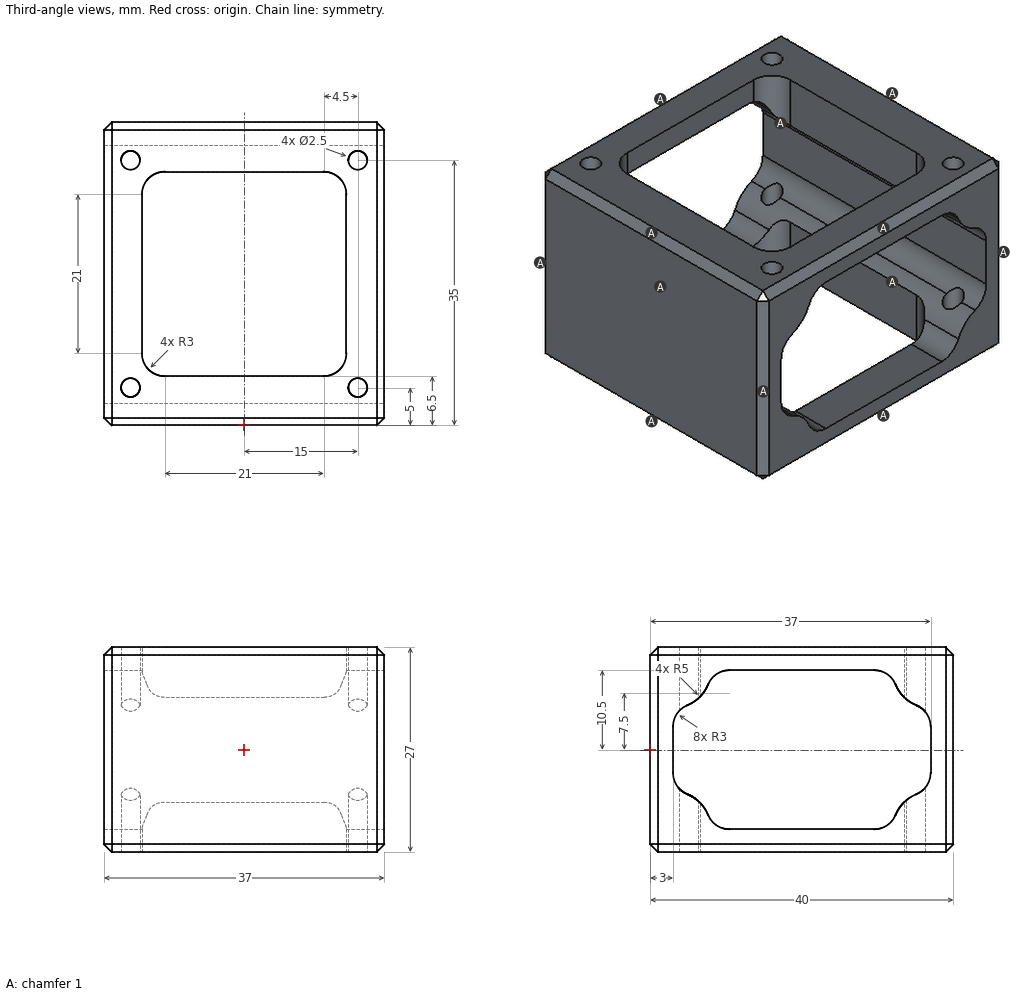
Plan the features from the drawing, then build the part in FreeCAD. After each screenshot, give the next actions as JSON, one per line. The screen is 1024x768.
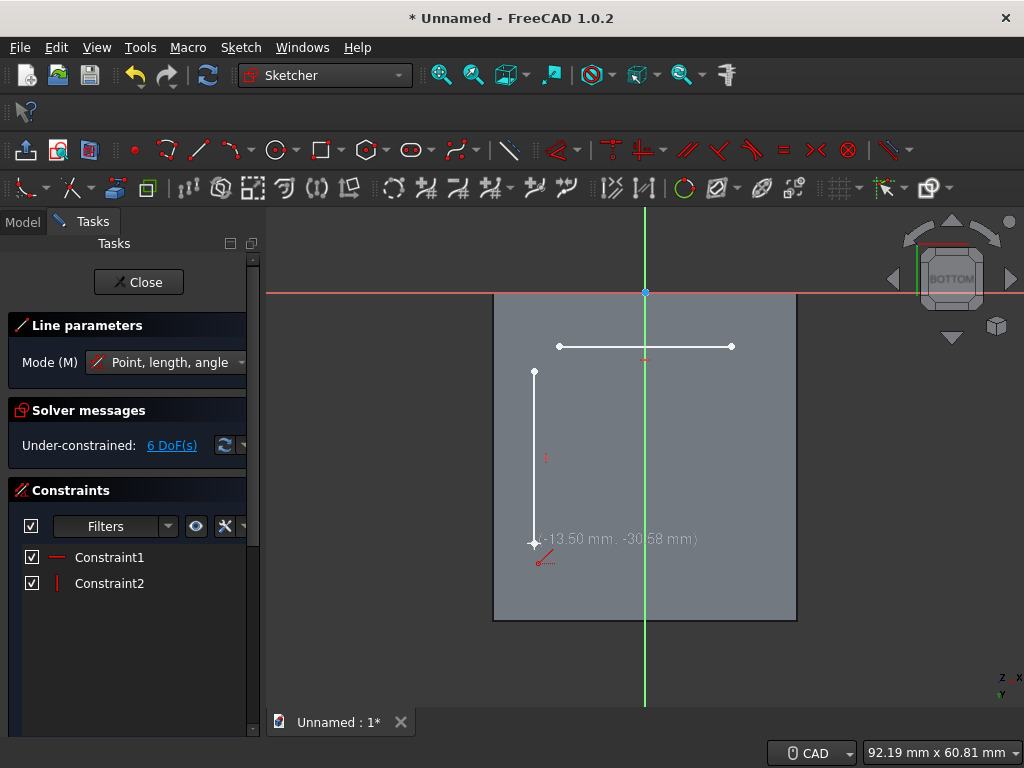
{"action": "left_click", "coordinate": [559, 568]}
{"action": "left_click", "coordinate": [731, 568]}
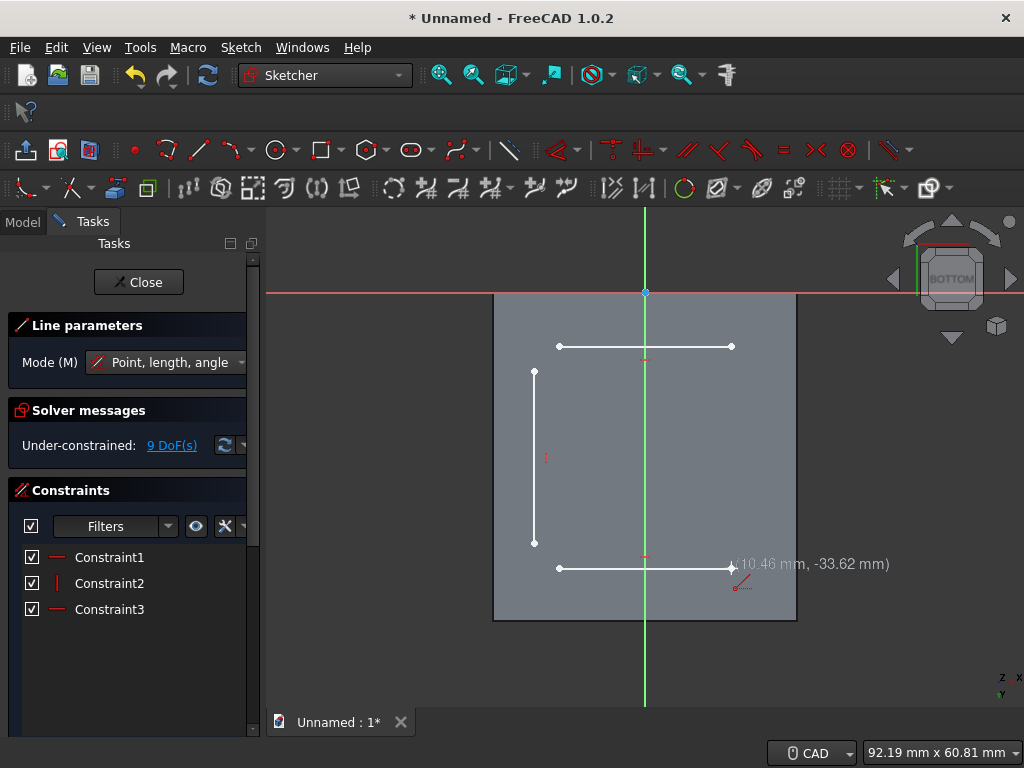
{"action": "left_click", "coordinate": [756, 543]}
{"action": "left_click", "coordinate": [756, 371]}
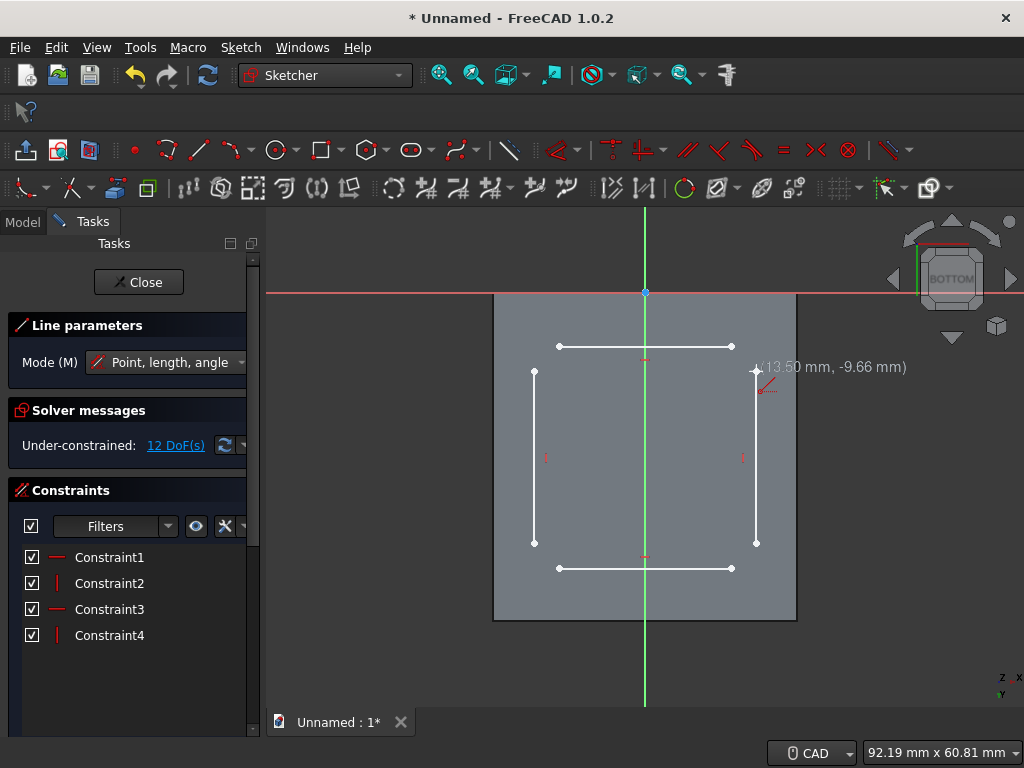
{"action": "key", "text": "g 3 a"}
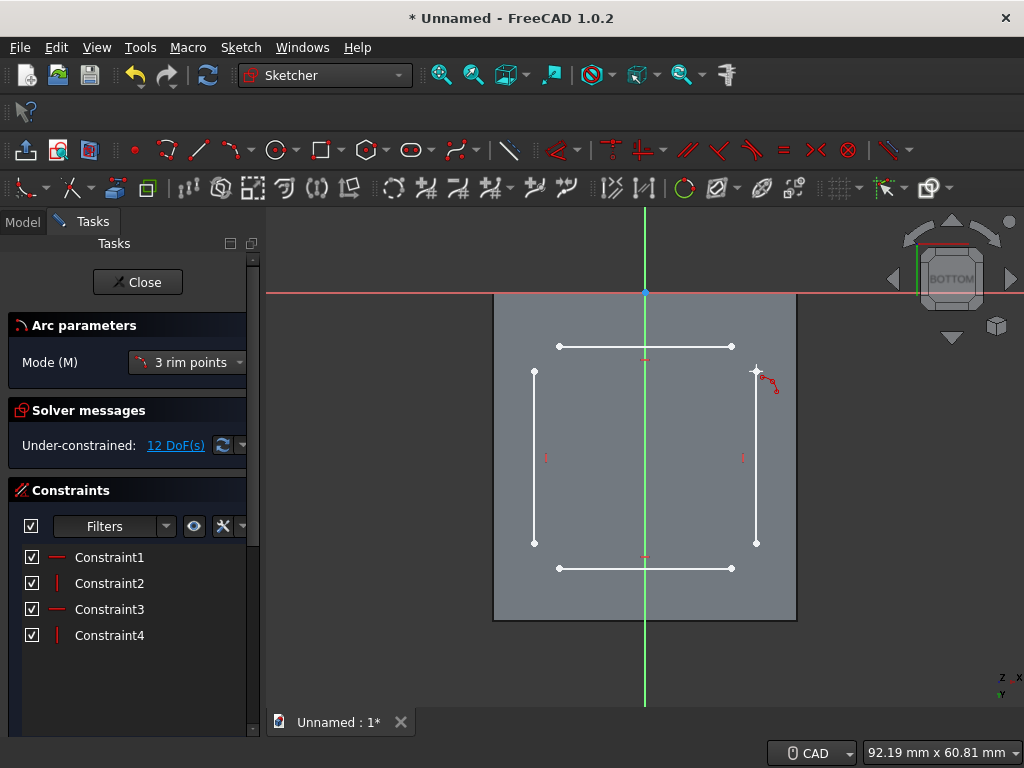
{"action": "left_click", "coordinate": [559, 347]}
{"action": "left_click", "coordinate": [534, 372]}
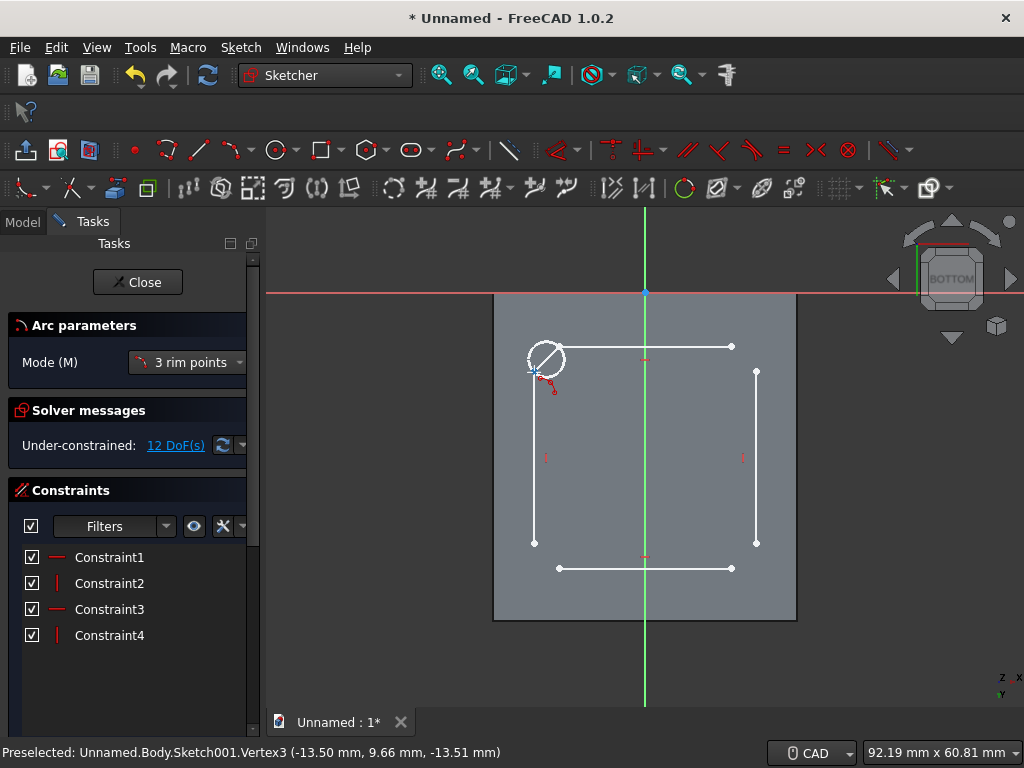
{"action": "scroll", "coordinate": [541, 353], "scroll_direction": "up", "scroll_amount": 4}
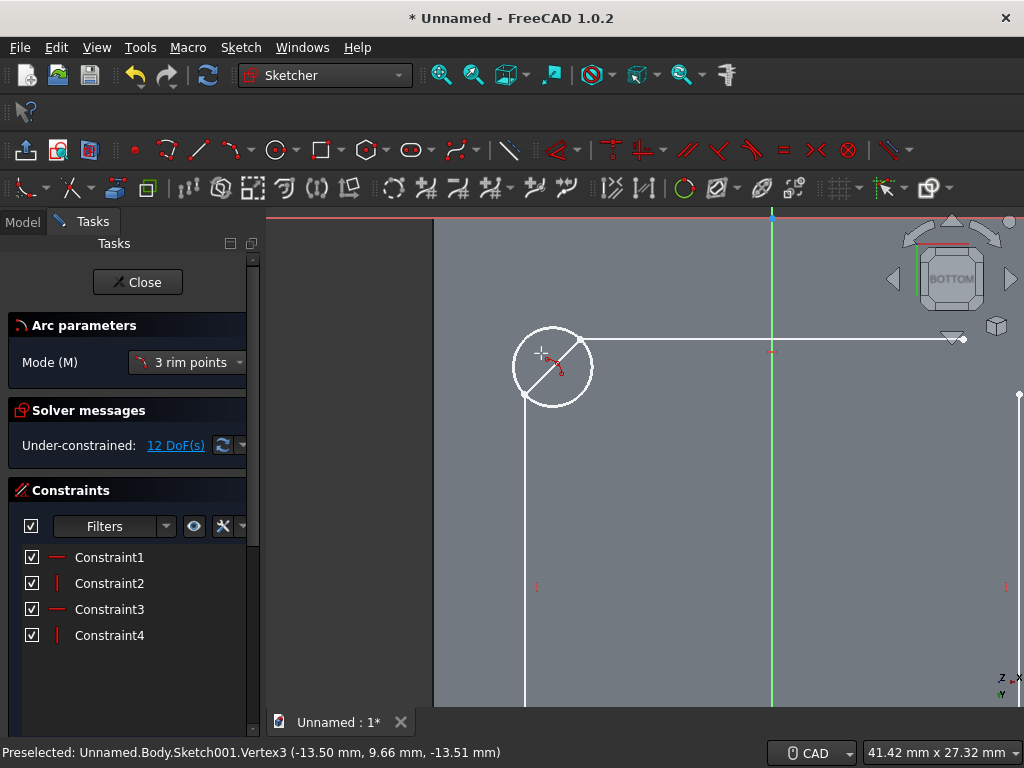
{"action": "left_click", "coordinate": [541, 353]}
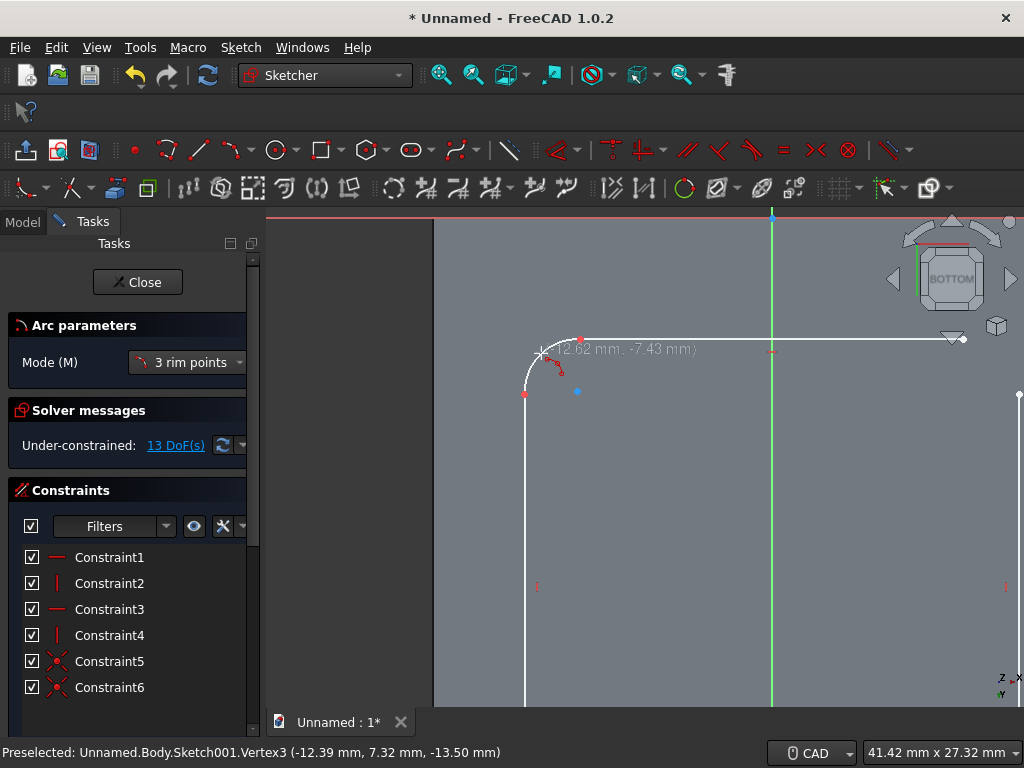
{"action": "scroll", "coordinate": [417, 381], "scroll_direction": "down", "scroll_amount": 4}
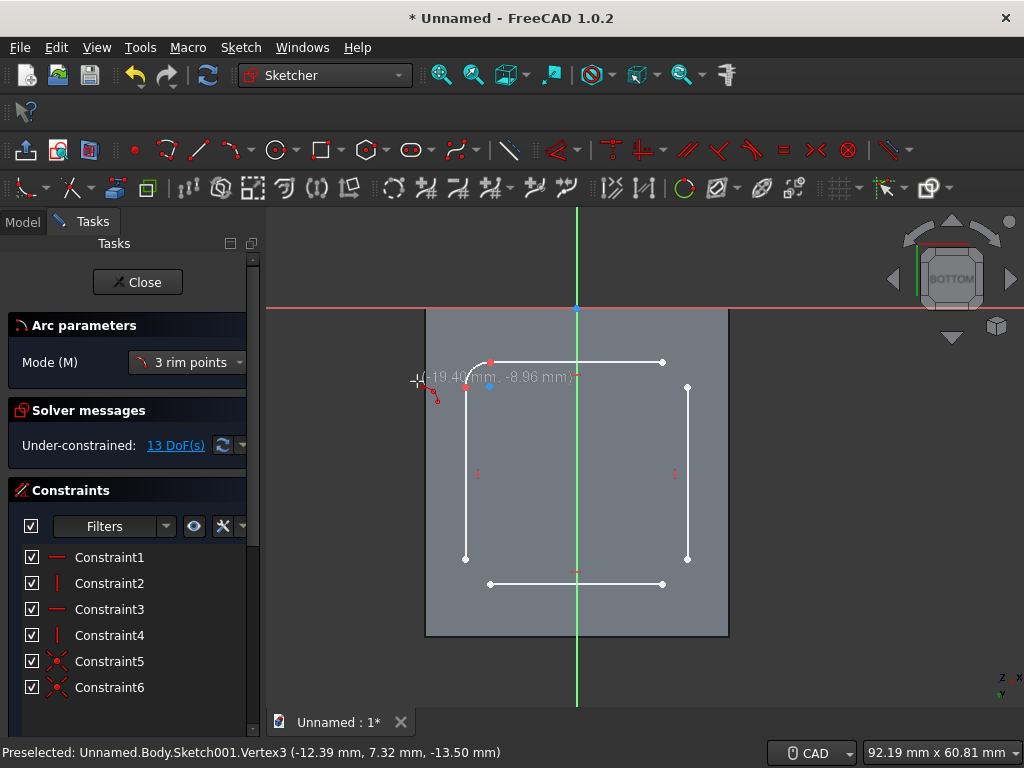
{"action": "left_click", "coordinate": [466, 559]}
{"action": "left_click", "coordinate": [491, 584]}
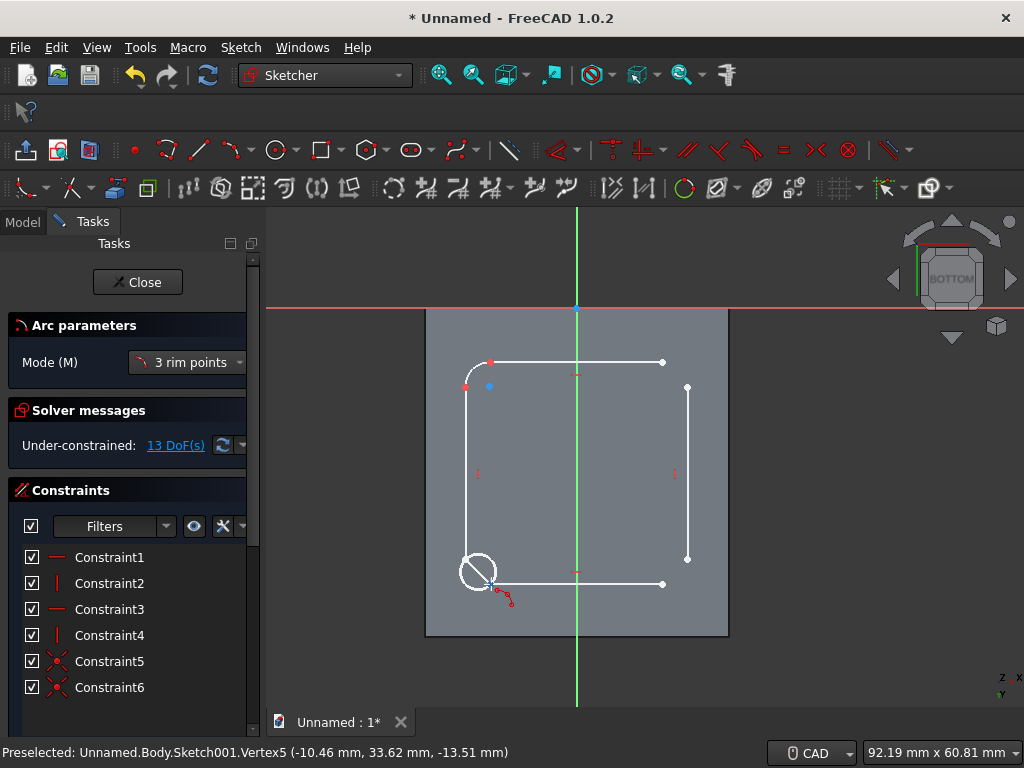
{"action": "scroll", "coordinate": [473, 576], "scroll_direction": "up", "scroll_amount": 4}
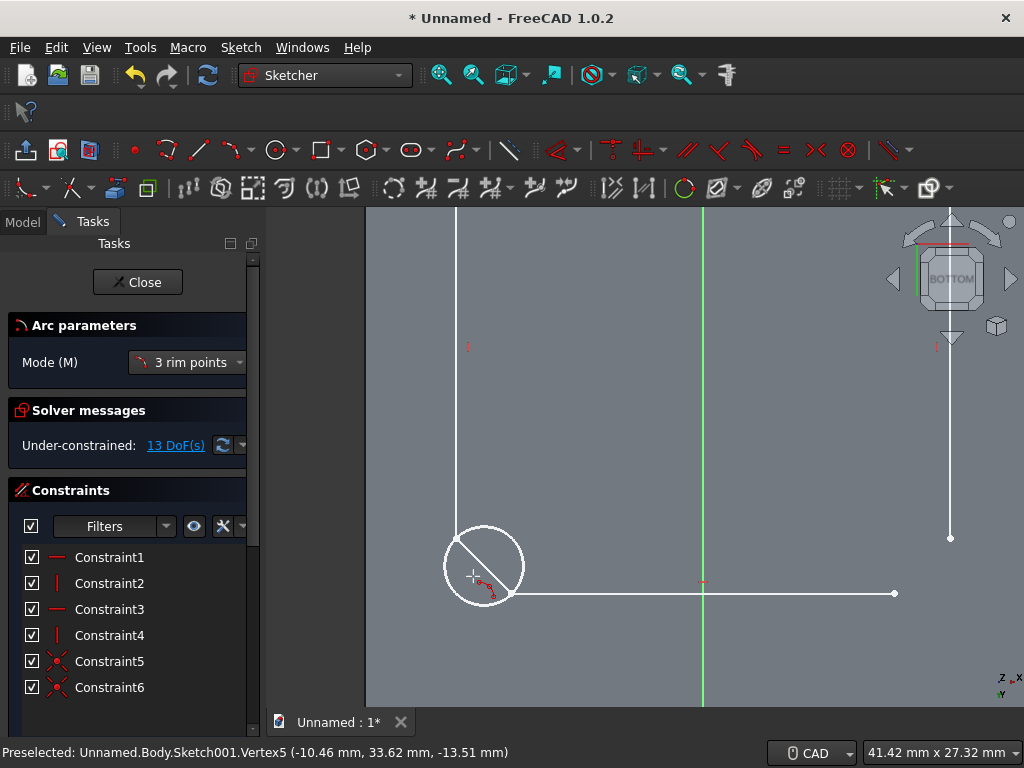
{"action": "left_click", "coordinate": [472, 576]}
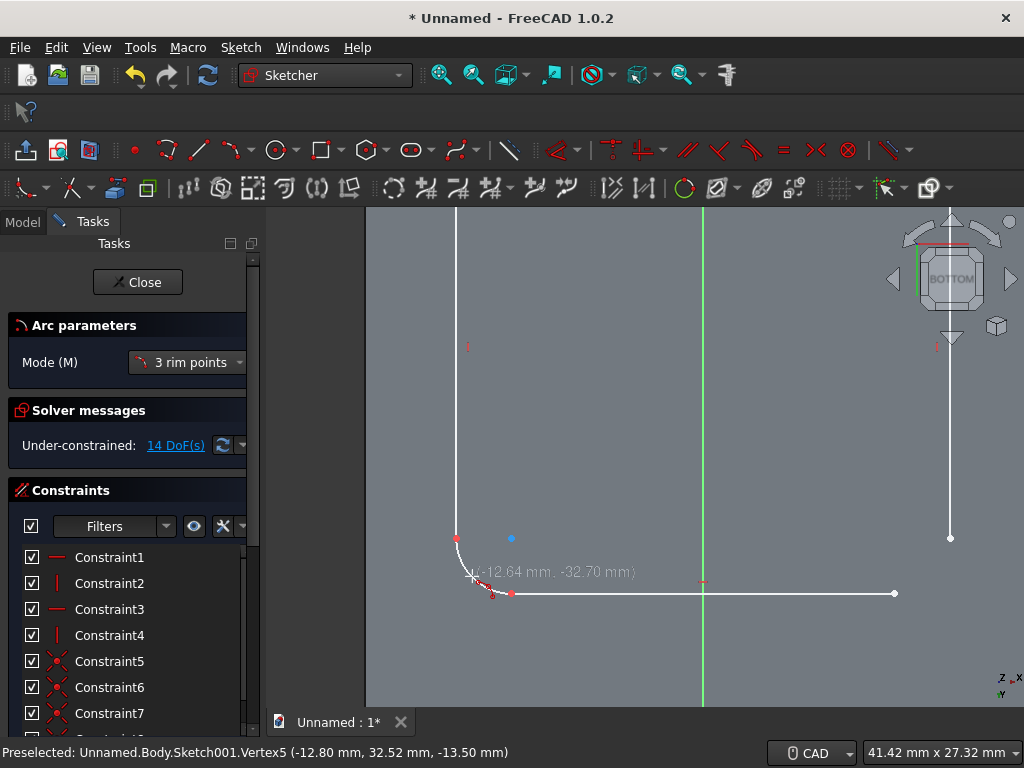
{"action": "scroll", "coordinate": [473, 577], "scroll_direction": "down", "scroll_amount": 4}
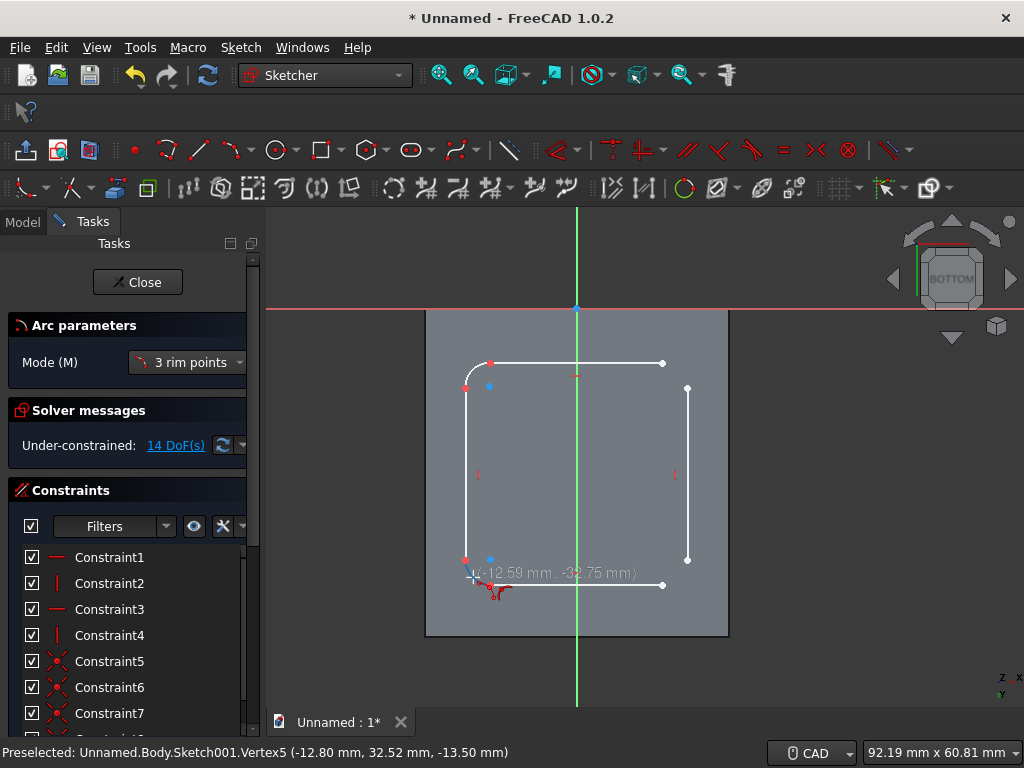
{"action": "left_click", "coordinate": [663, 585]}
{"action": "left_click", "coordinate": [688, 560]}